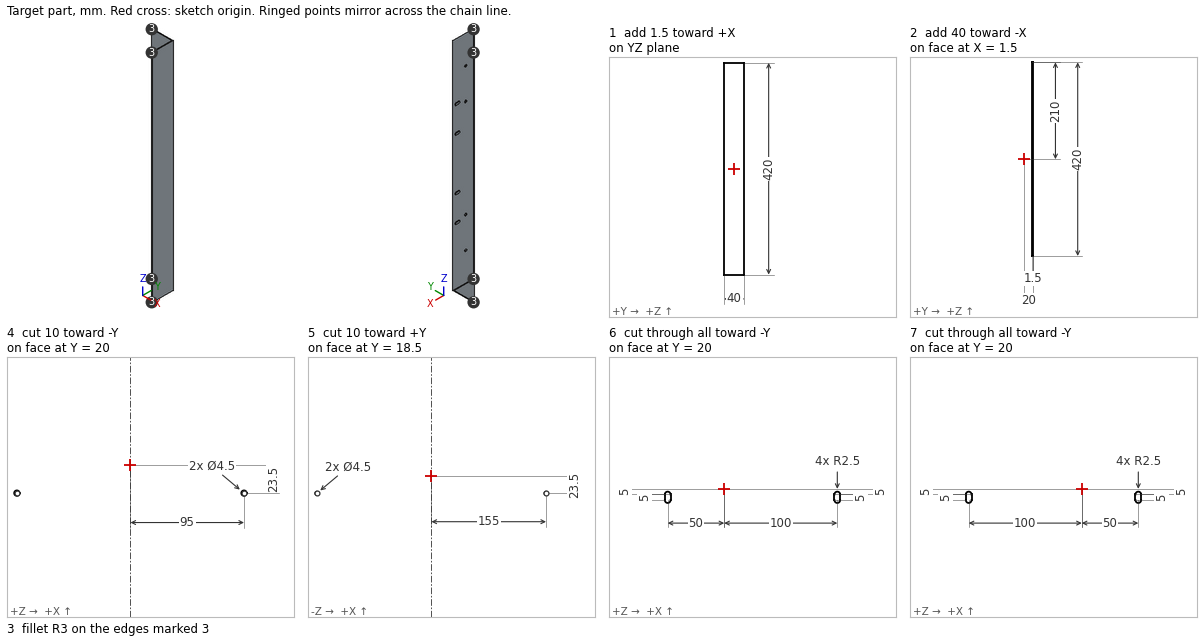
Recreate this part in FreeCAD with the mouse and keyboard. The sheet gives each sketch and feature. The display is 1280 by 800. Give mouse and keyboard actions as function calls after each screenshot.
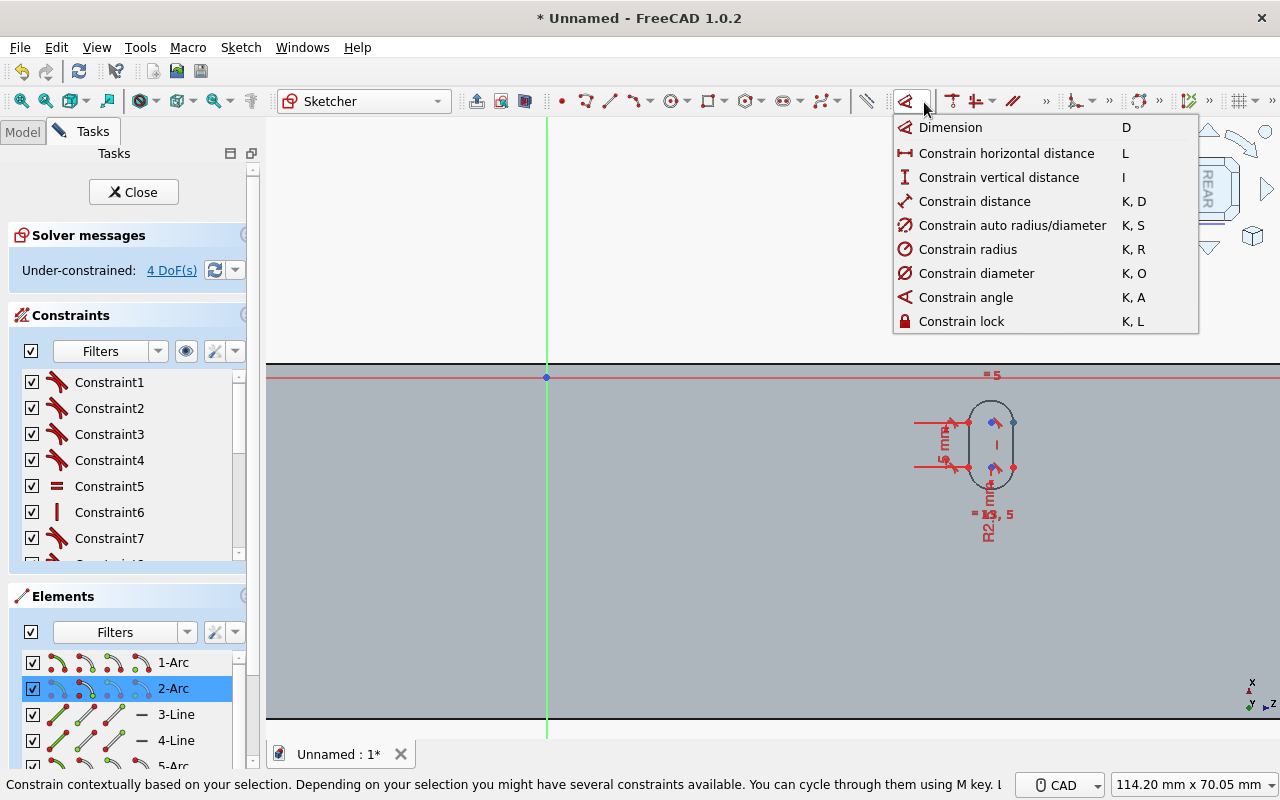
click(1046, 177)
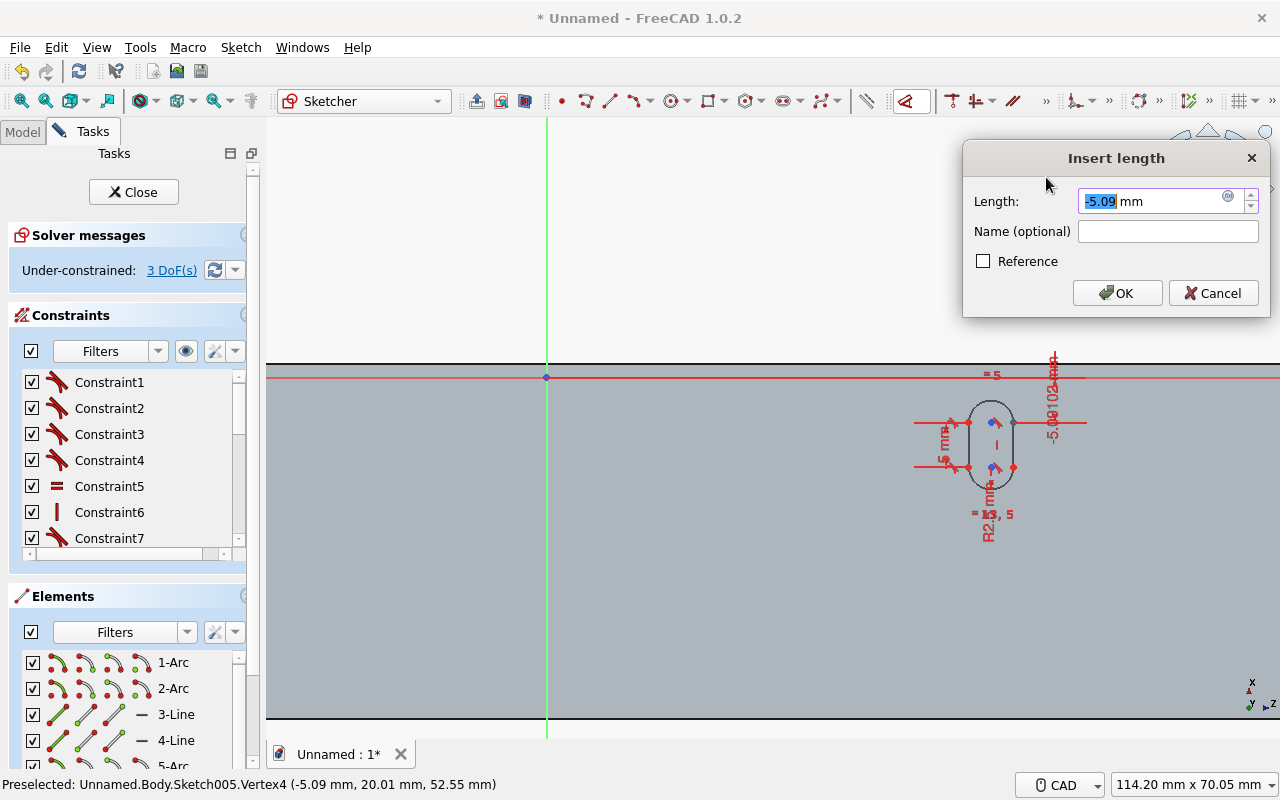
text(-5)
key(Return)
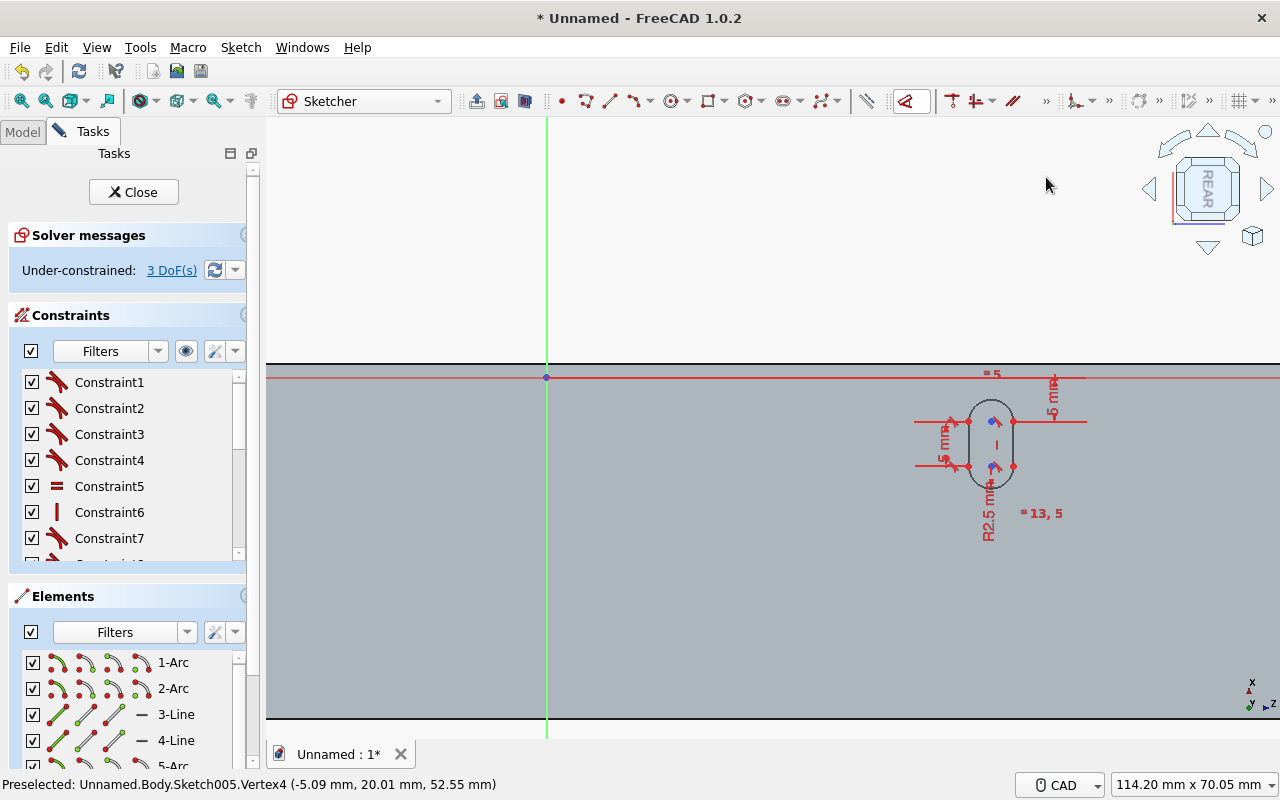
scroll(1014, 424, down, 4)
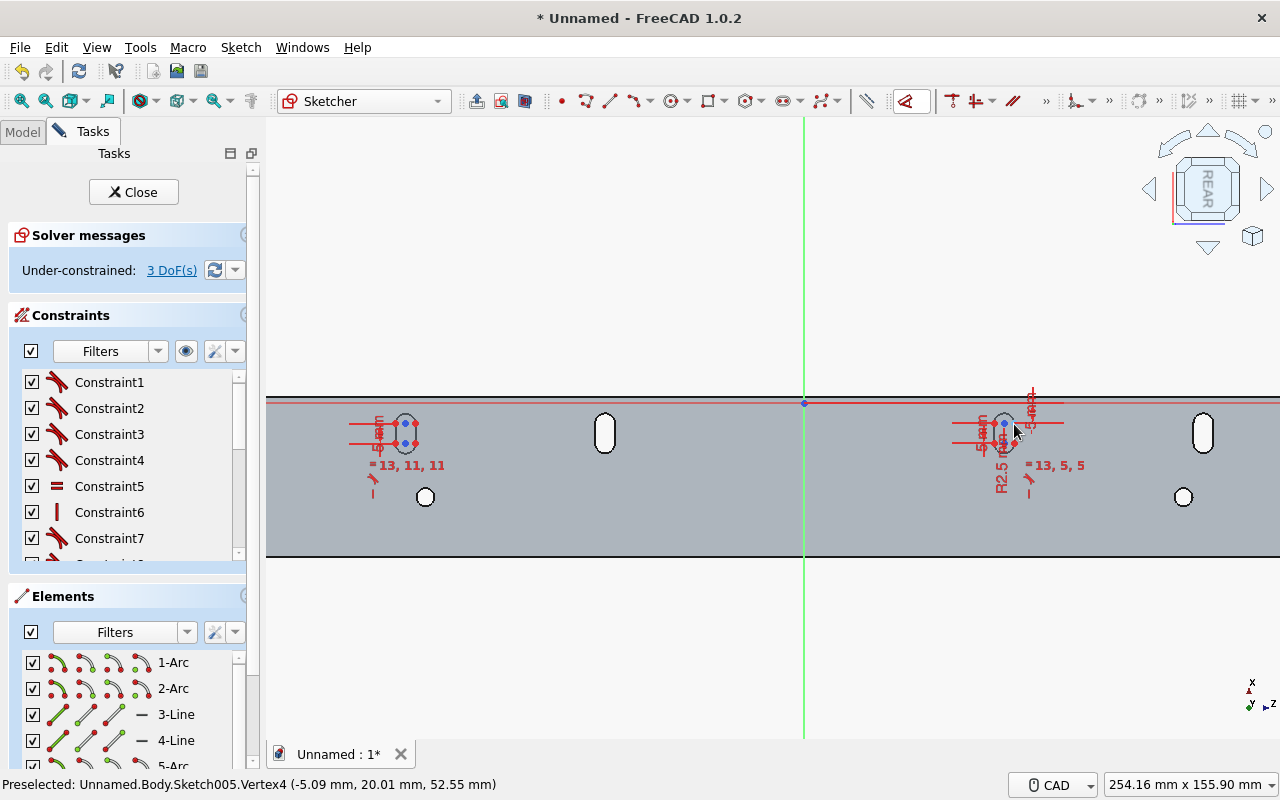
scroll(416, 424, up, 4)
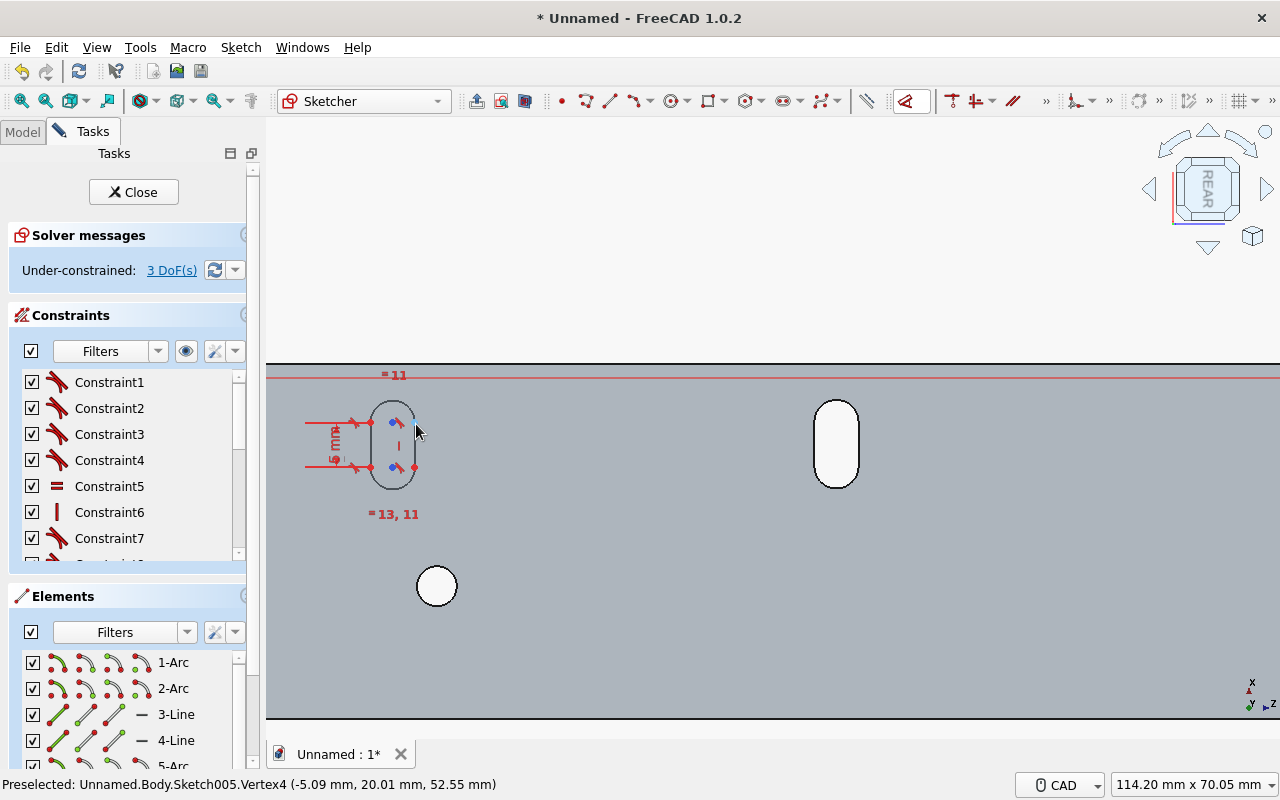
click(415, 423)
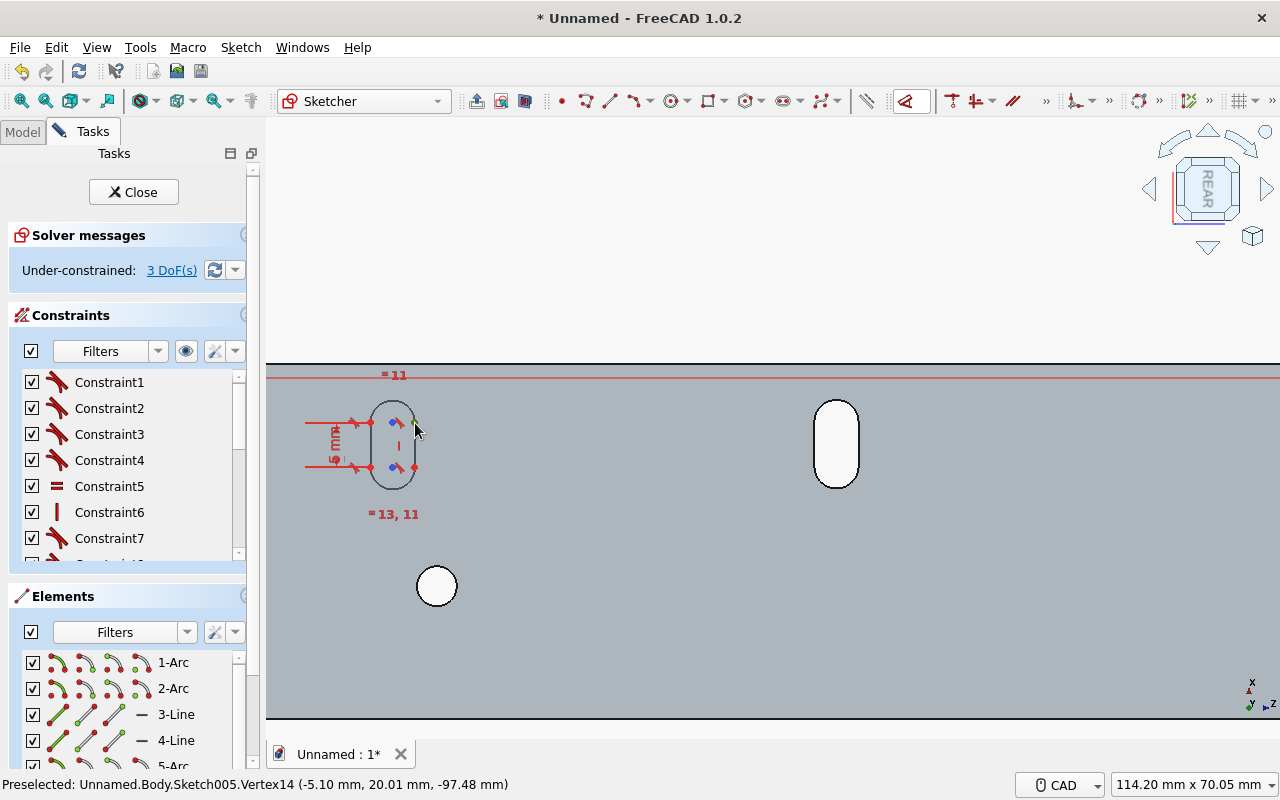
click(924, 102)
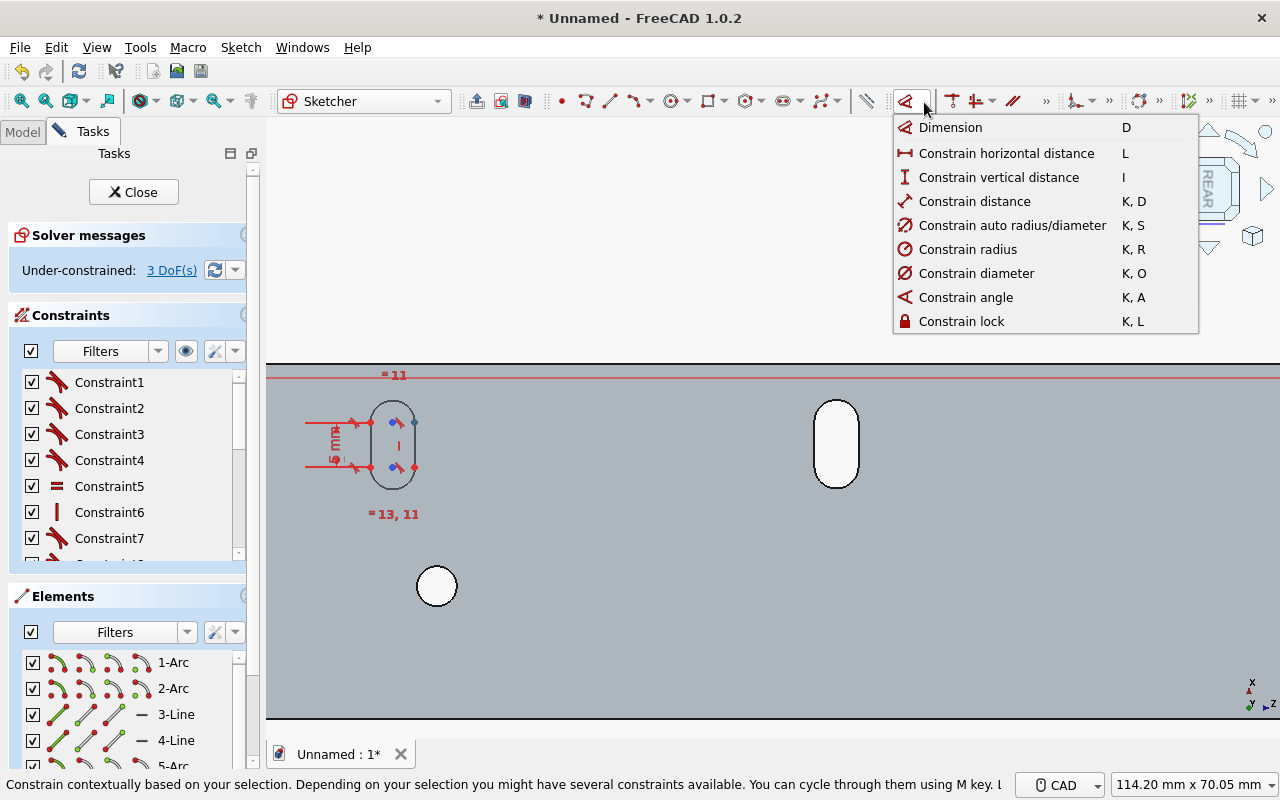
click(1046, 177)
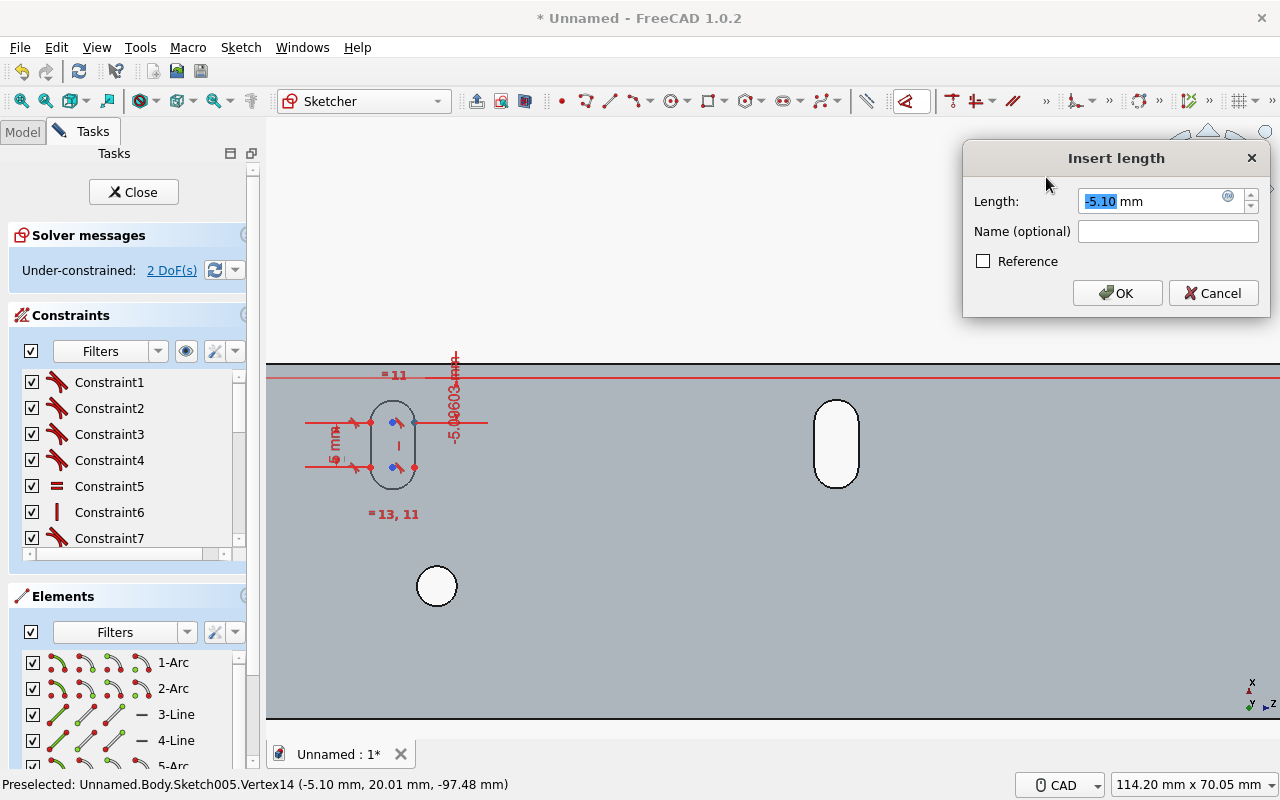
text(-5)
key(Return)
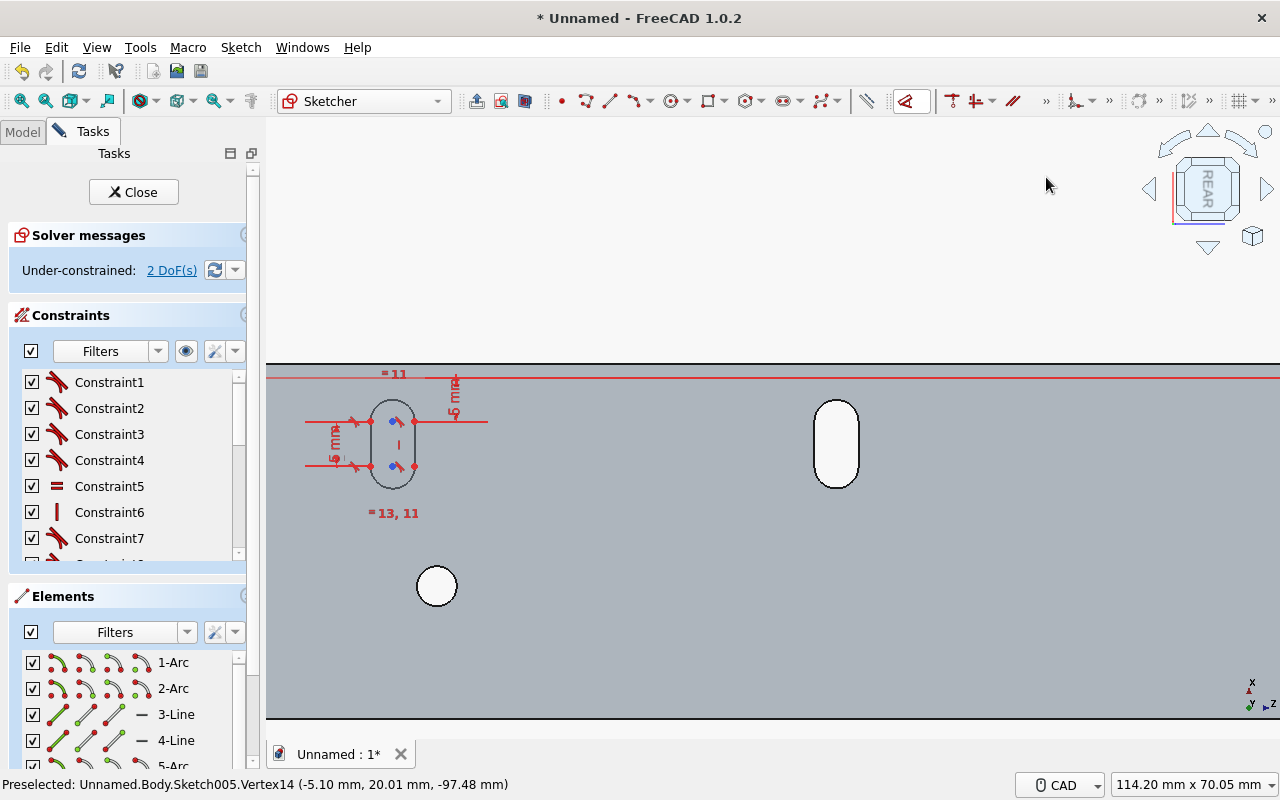
scroll(416, 424, down, 4)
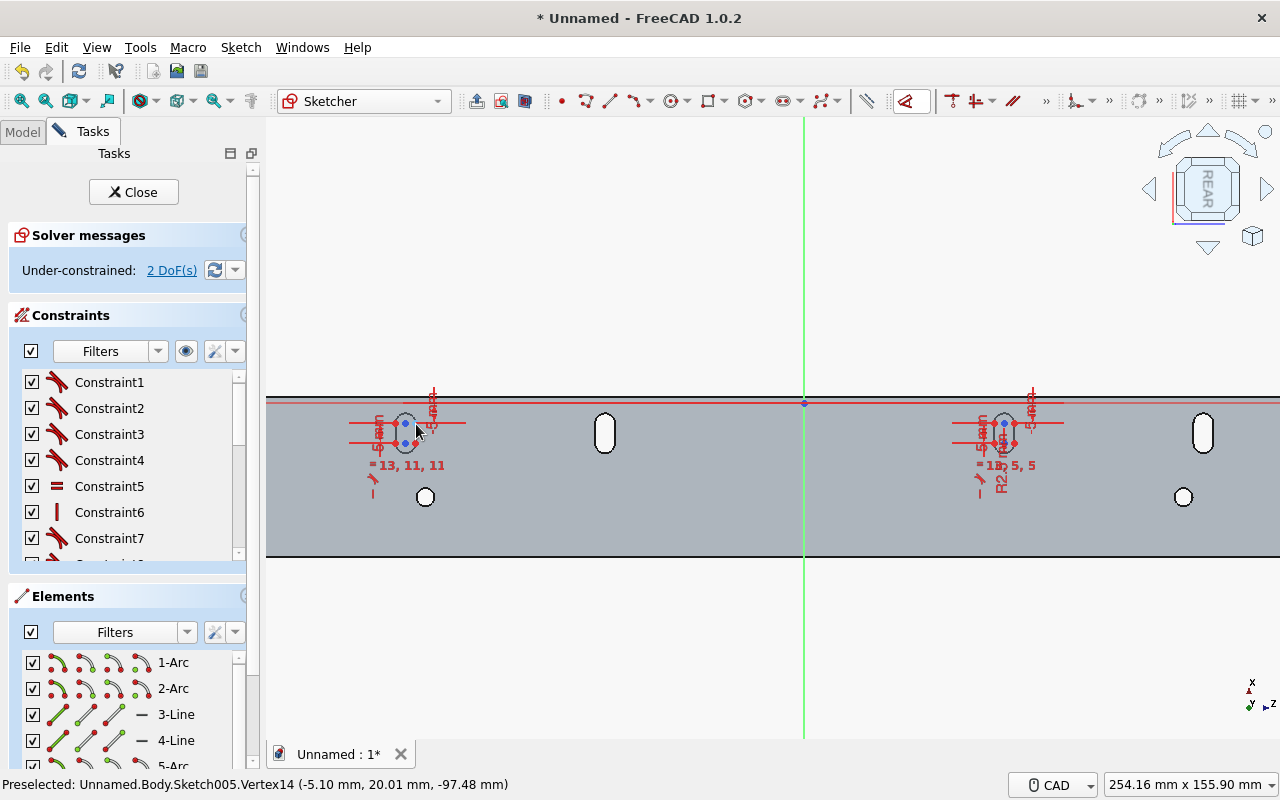
scroll(1004, 443, up, 2)